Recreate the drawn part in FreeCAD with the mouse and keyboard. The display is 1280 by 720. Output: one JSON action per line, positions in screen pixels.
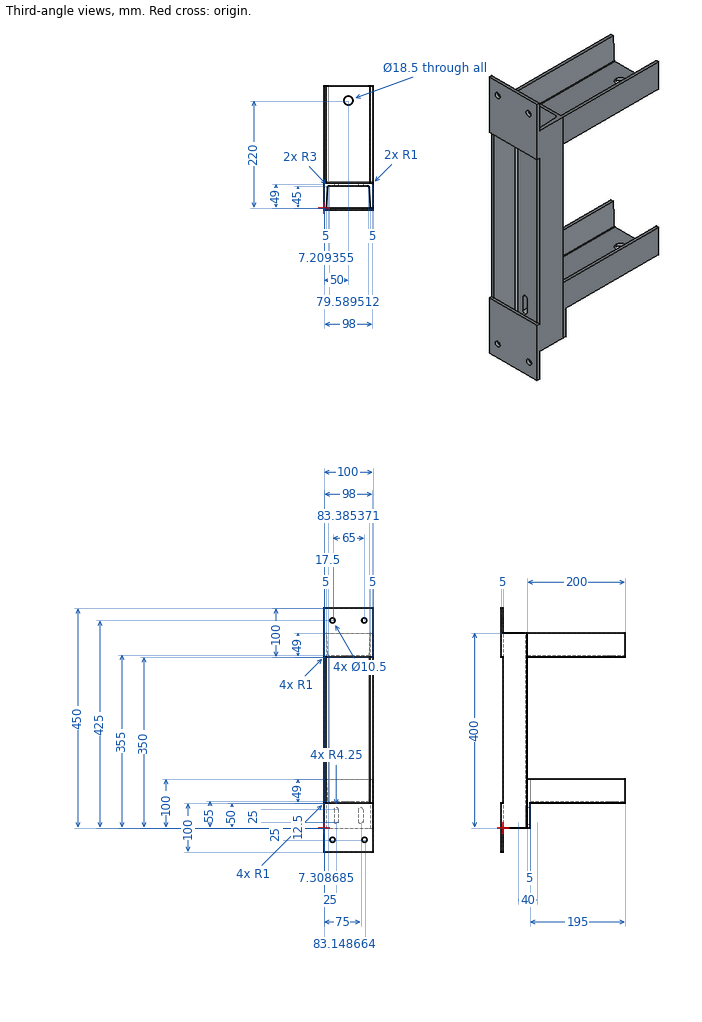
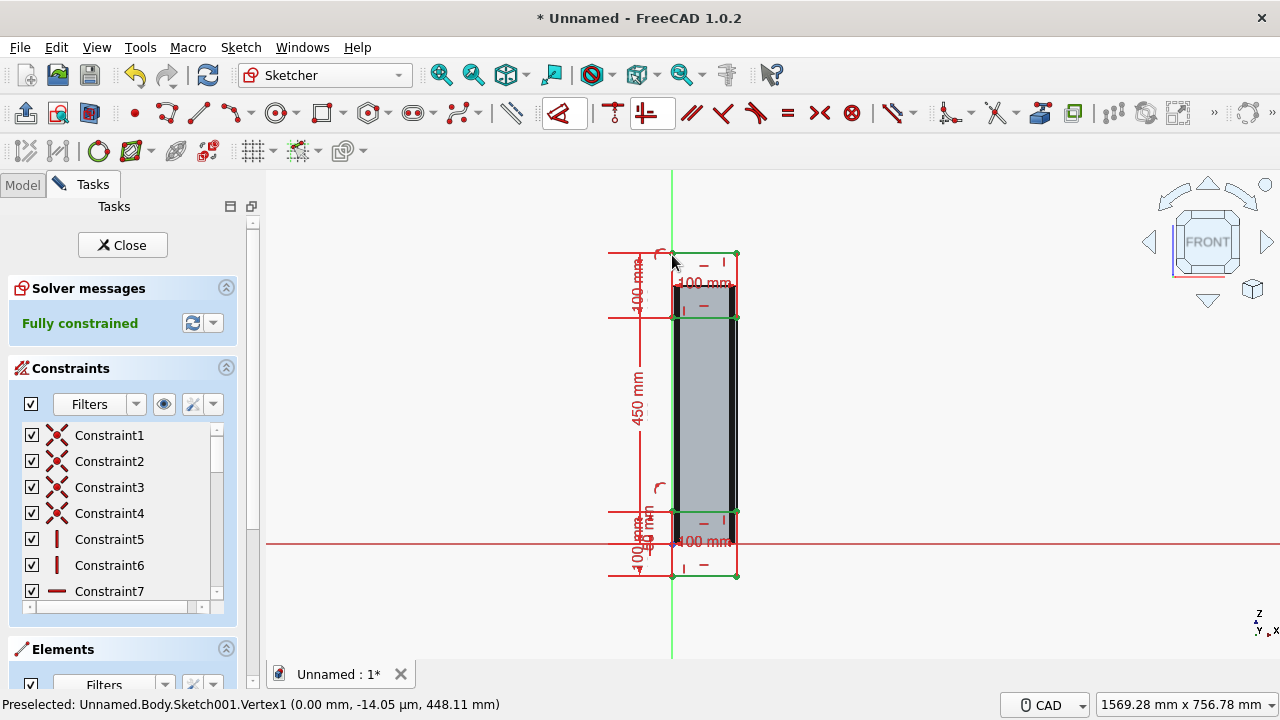
{"action": "left_click", "coordinate": [123, 245]}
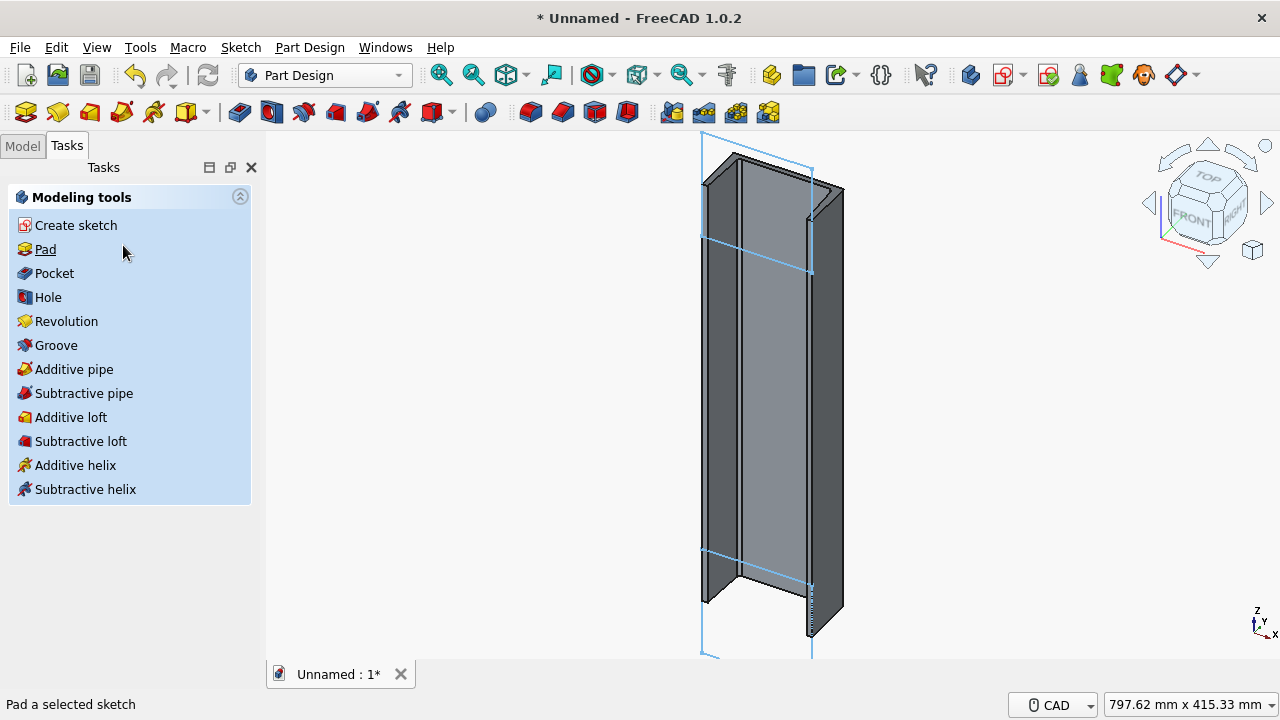
{"action": "left_click", "coordinate": [26, 112]}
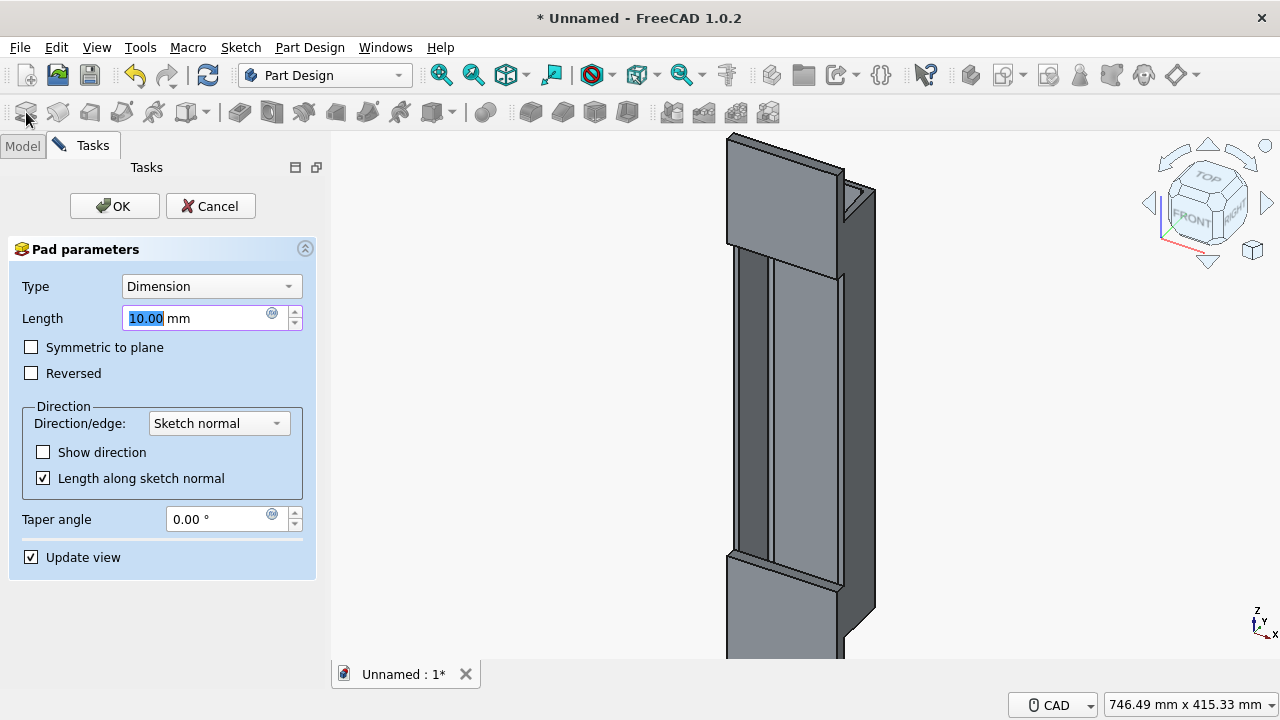
{"action": "type", "text": "5"}
{"action": "key", "text": "Tab"}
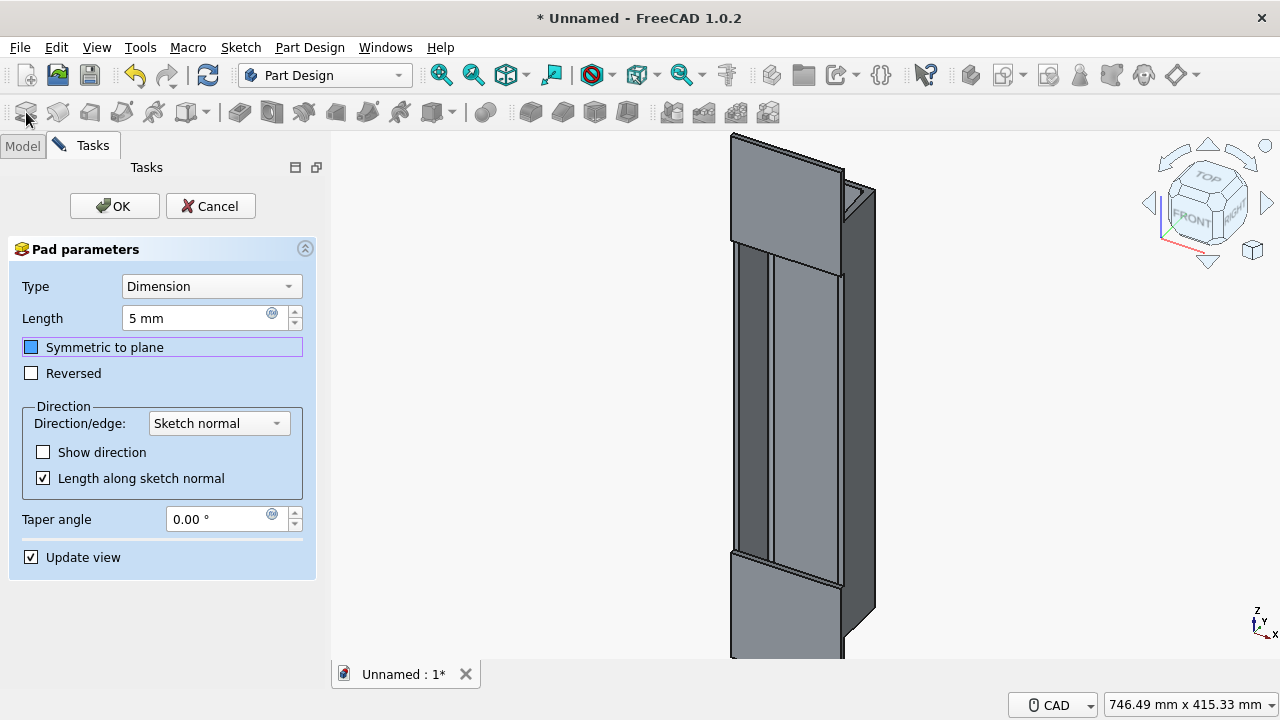
{"action": "left_click", "coordinate": [115, 206]}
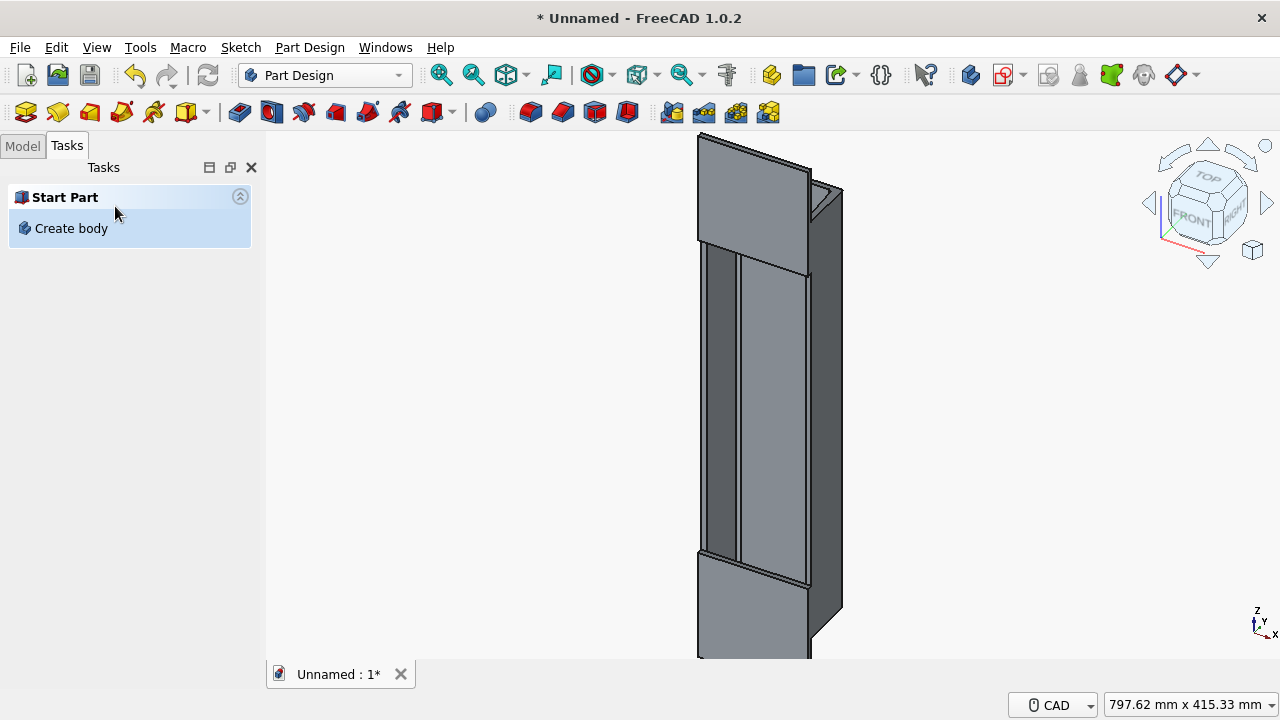
{"action": "key", "text": "v f"}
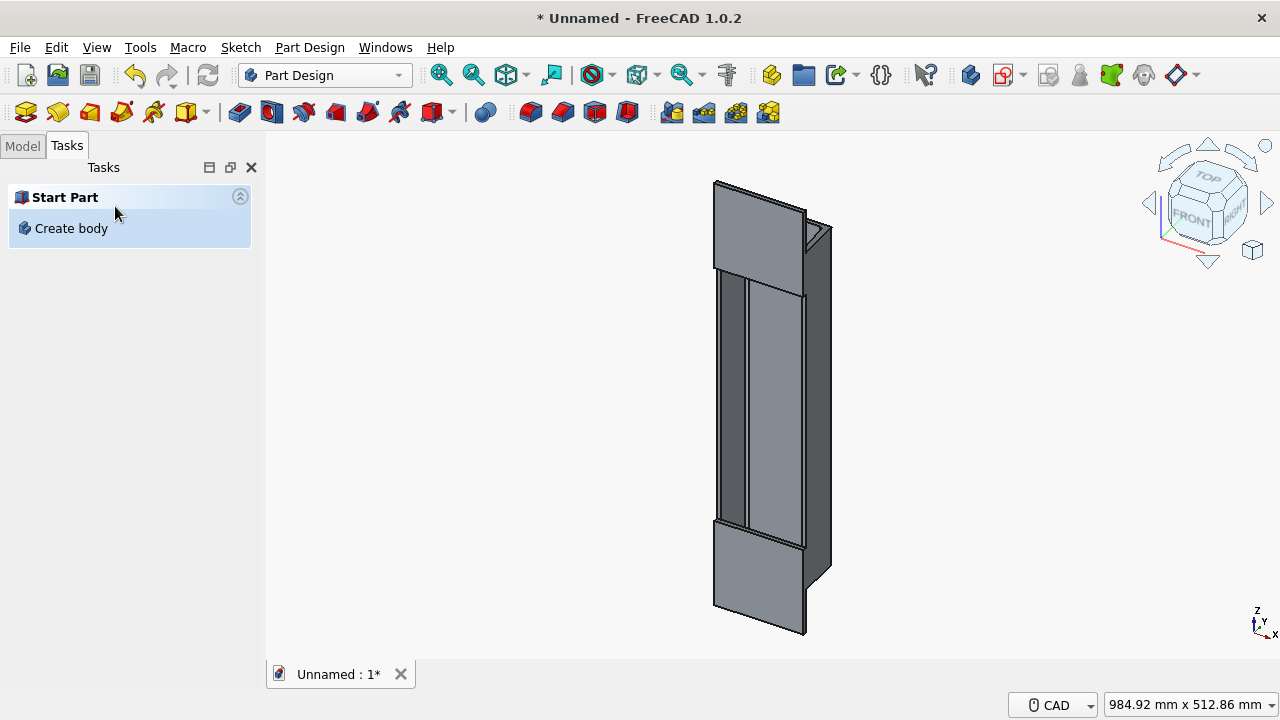
{"action": "left_click", "coordinate": [1004, 76]}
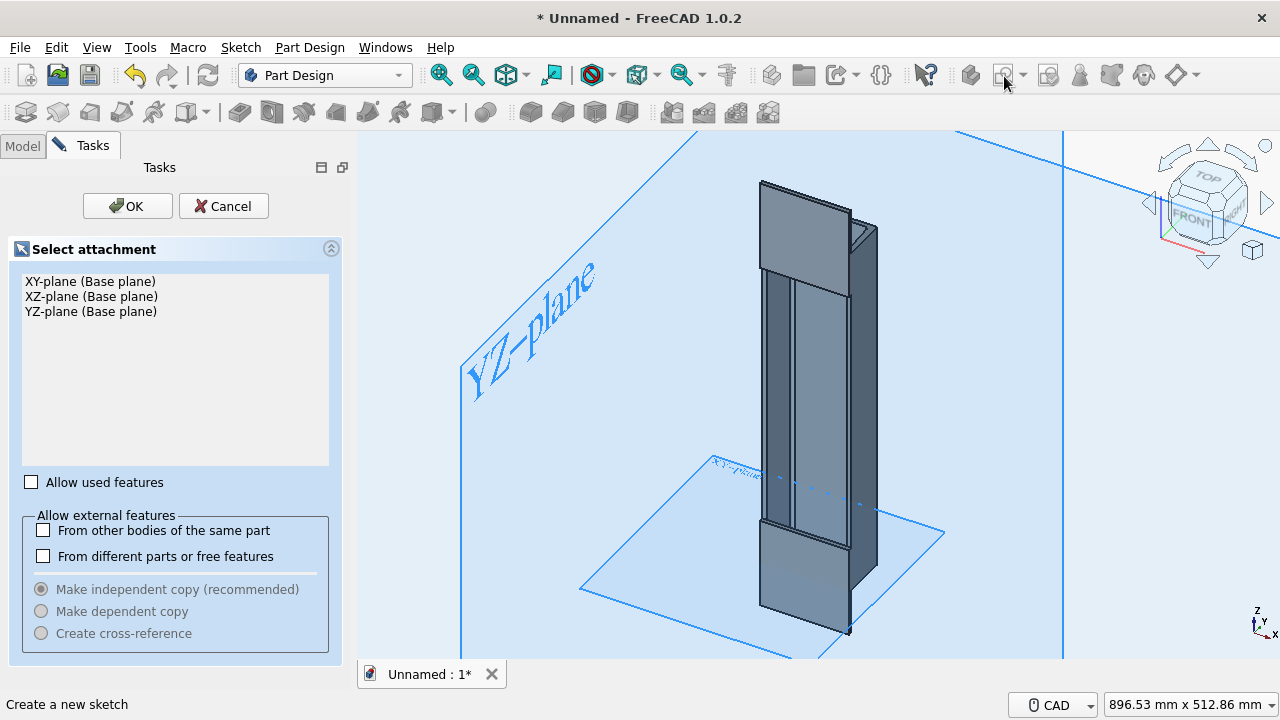
{"action": "left_click", "coordinate": [82, 296]}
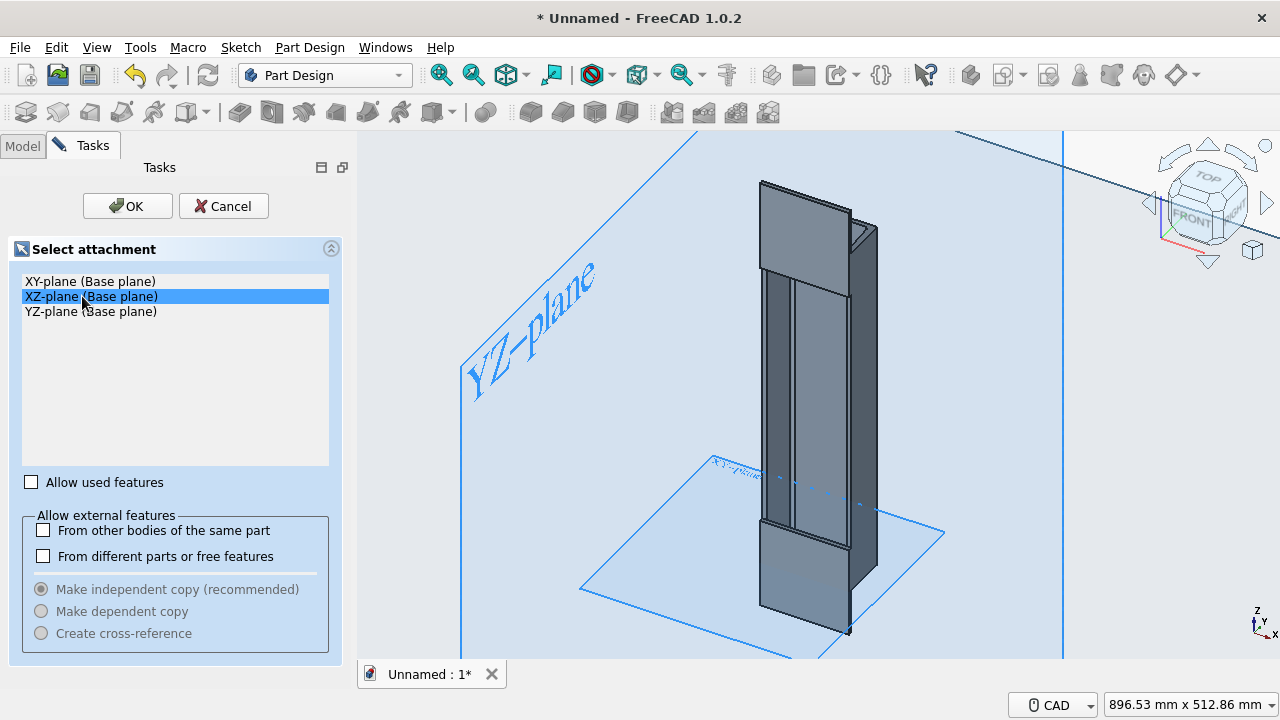
{"action": "left_click", "coordinate": [128, 206]}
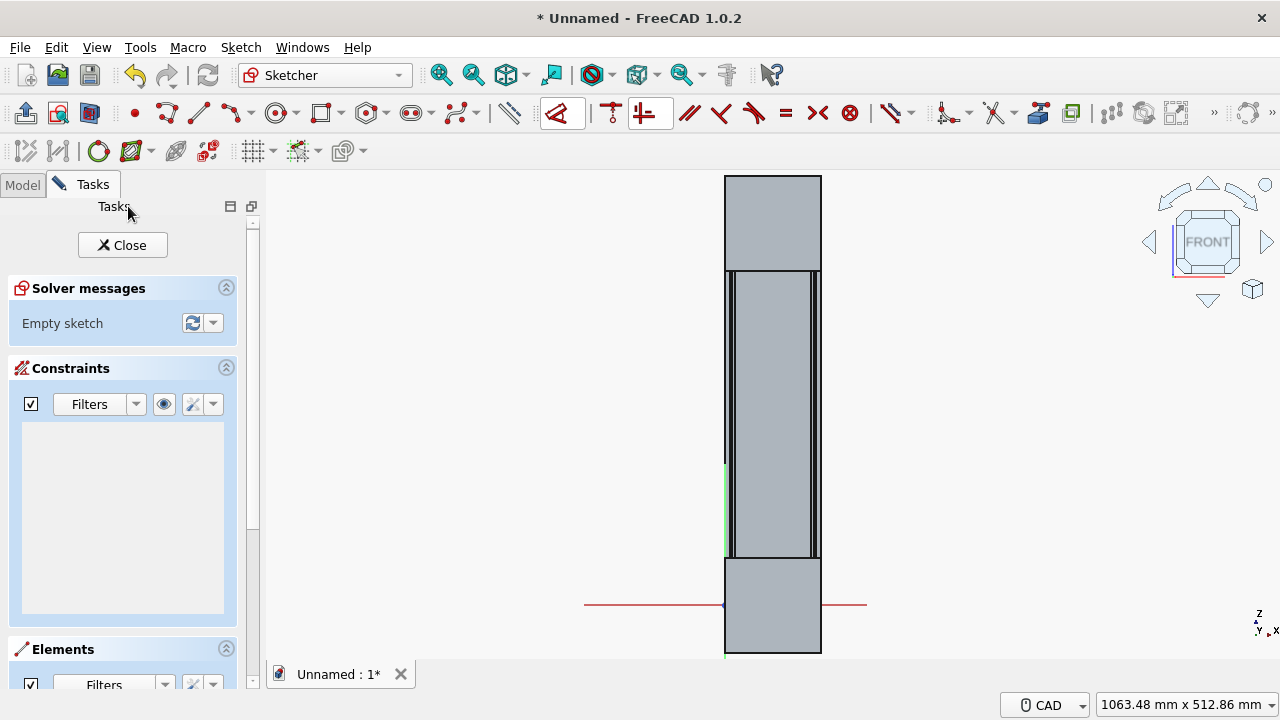
{"action": "left_click", "coordinate": [90, 114]}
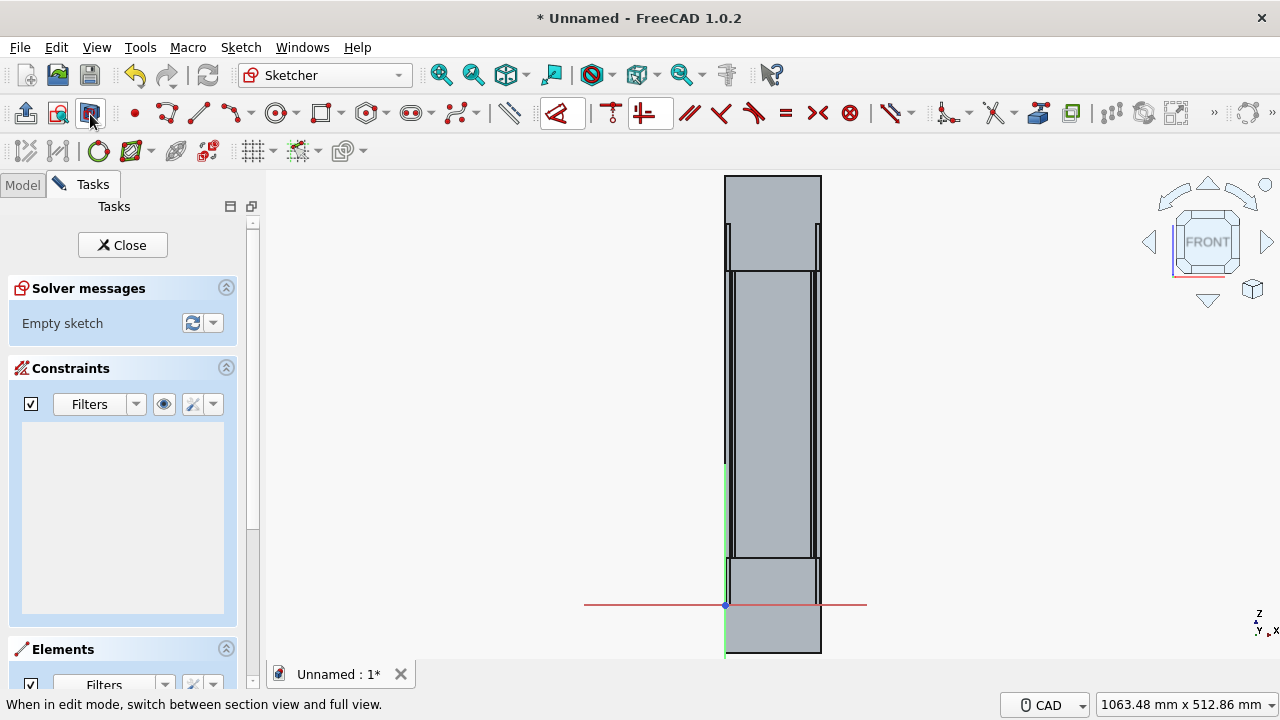
{"action": "scroll", "coordinate": [576, 415], "scroll_direction": "down", "scroll_amount": 2}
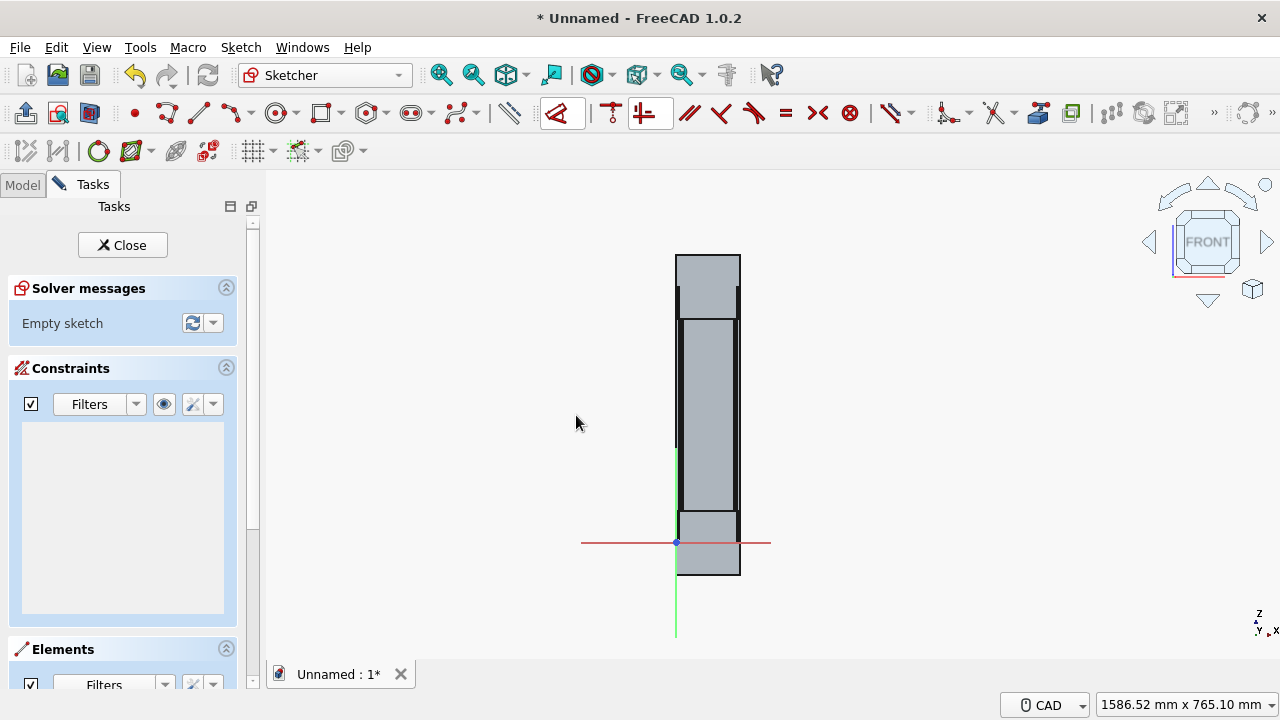
{"action": "left_click", "coordinate": [276, 114]}